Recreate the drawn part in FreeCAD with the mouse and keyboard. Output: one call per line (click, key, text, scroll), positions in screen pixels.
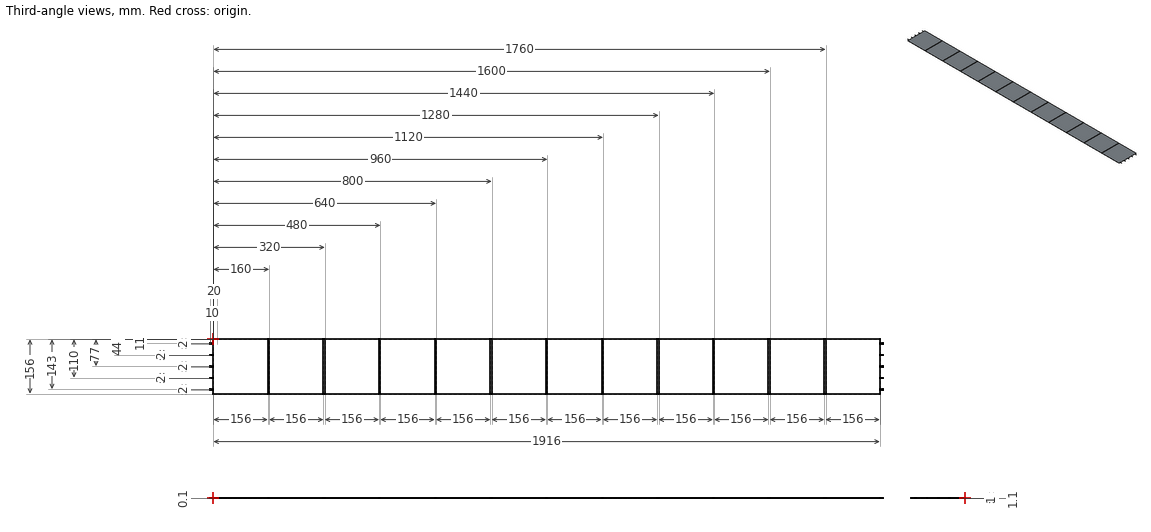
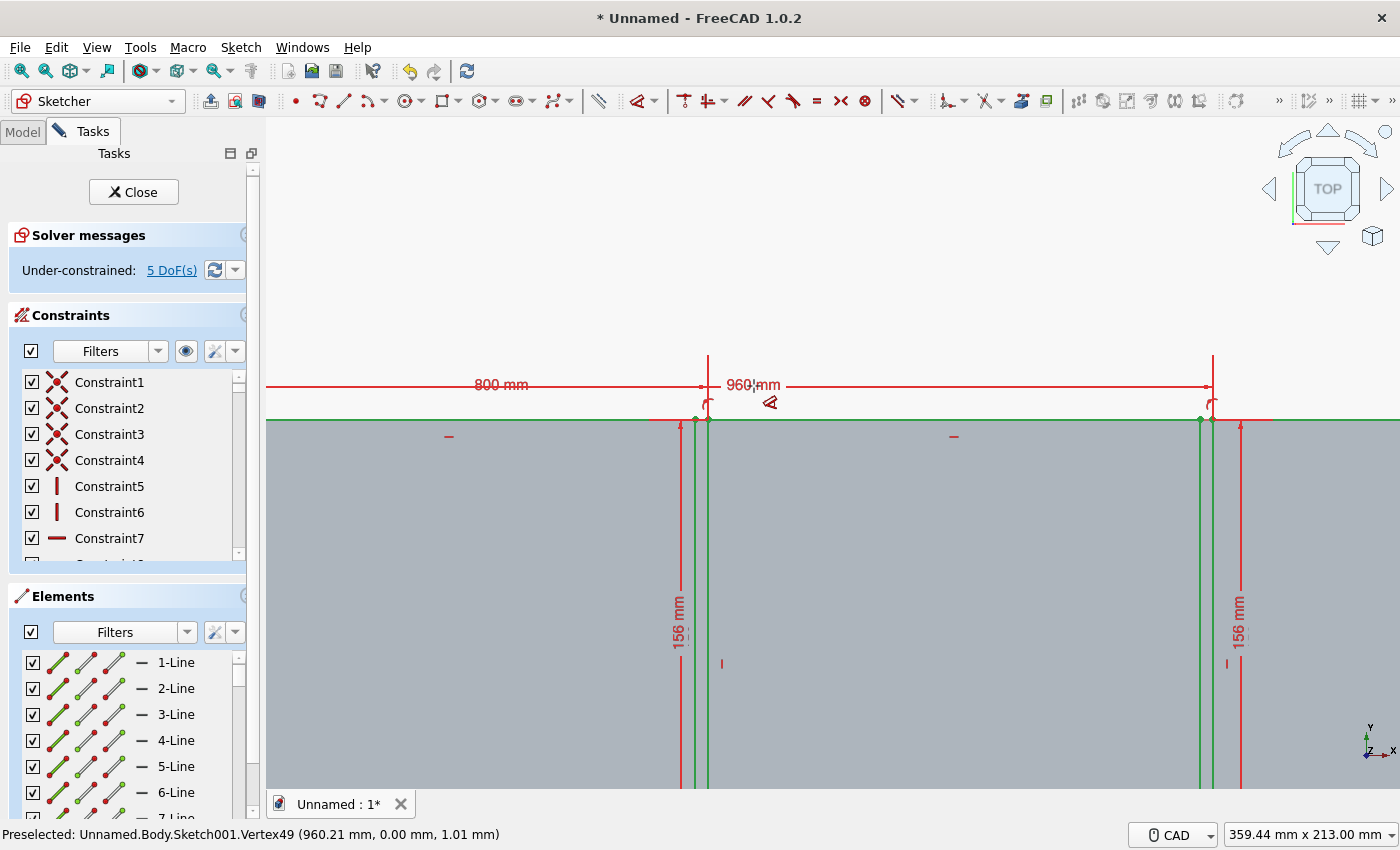
scroll(709, 426, down, 11)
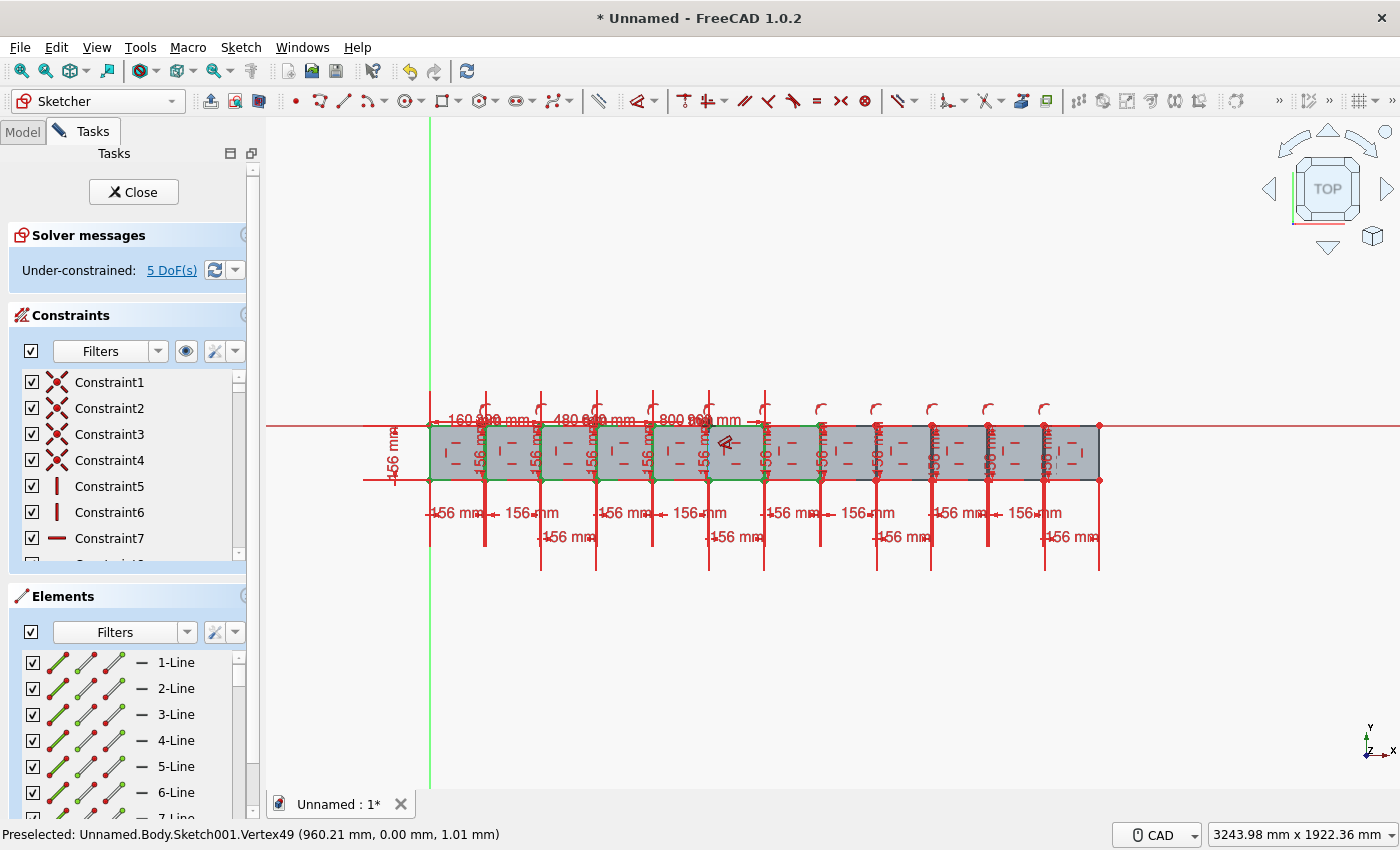
scroll(821, 426, up, 11)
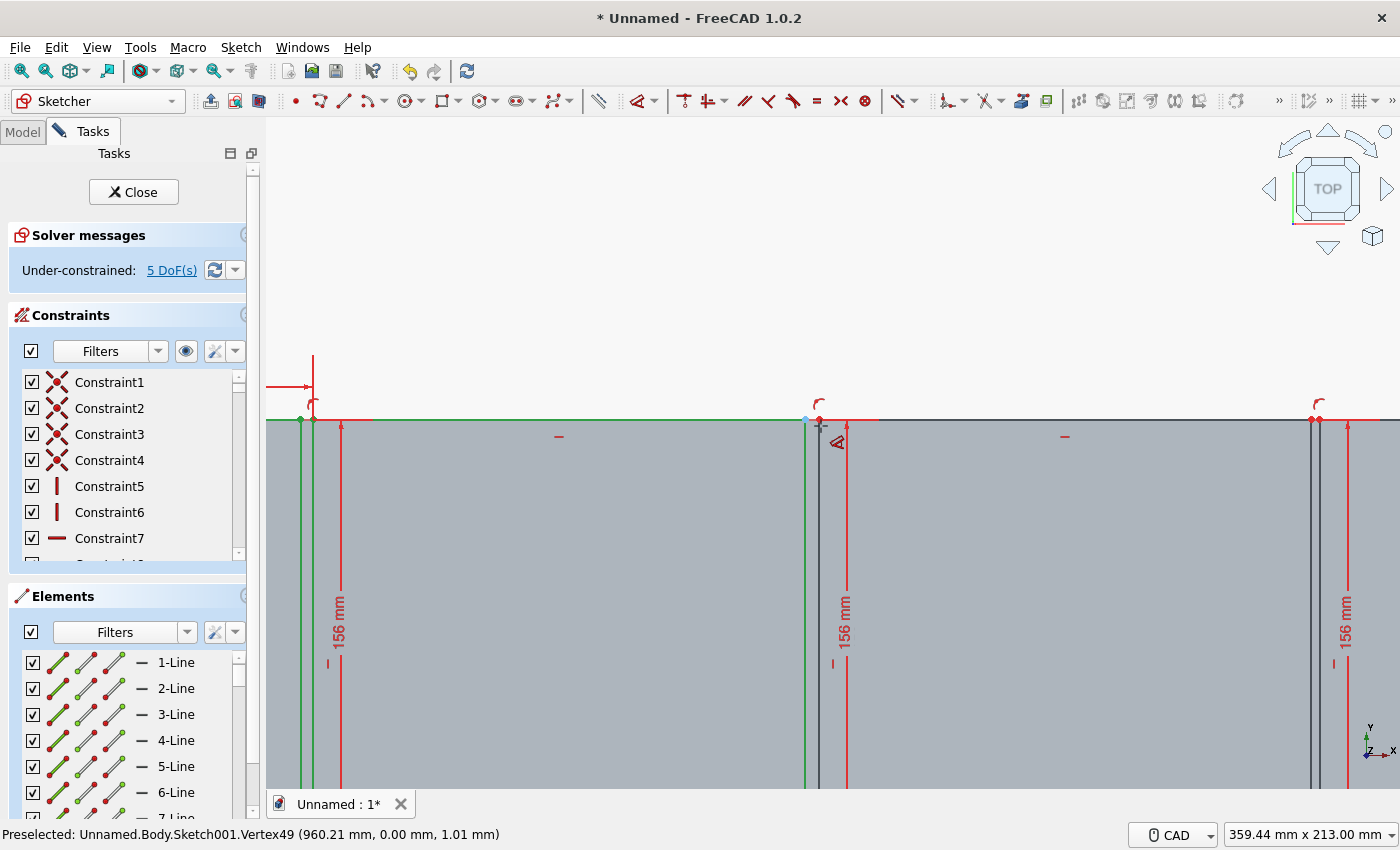
click(819, 420)
click(557, 386)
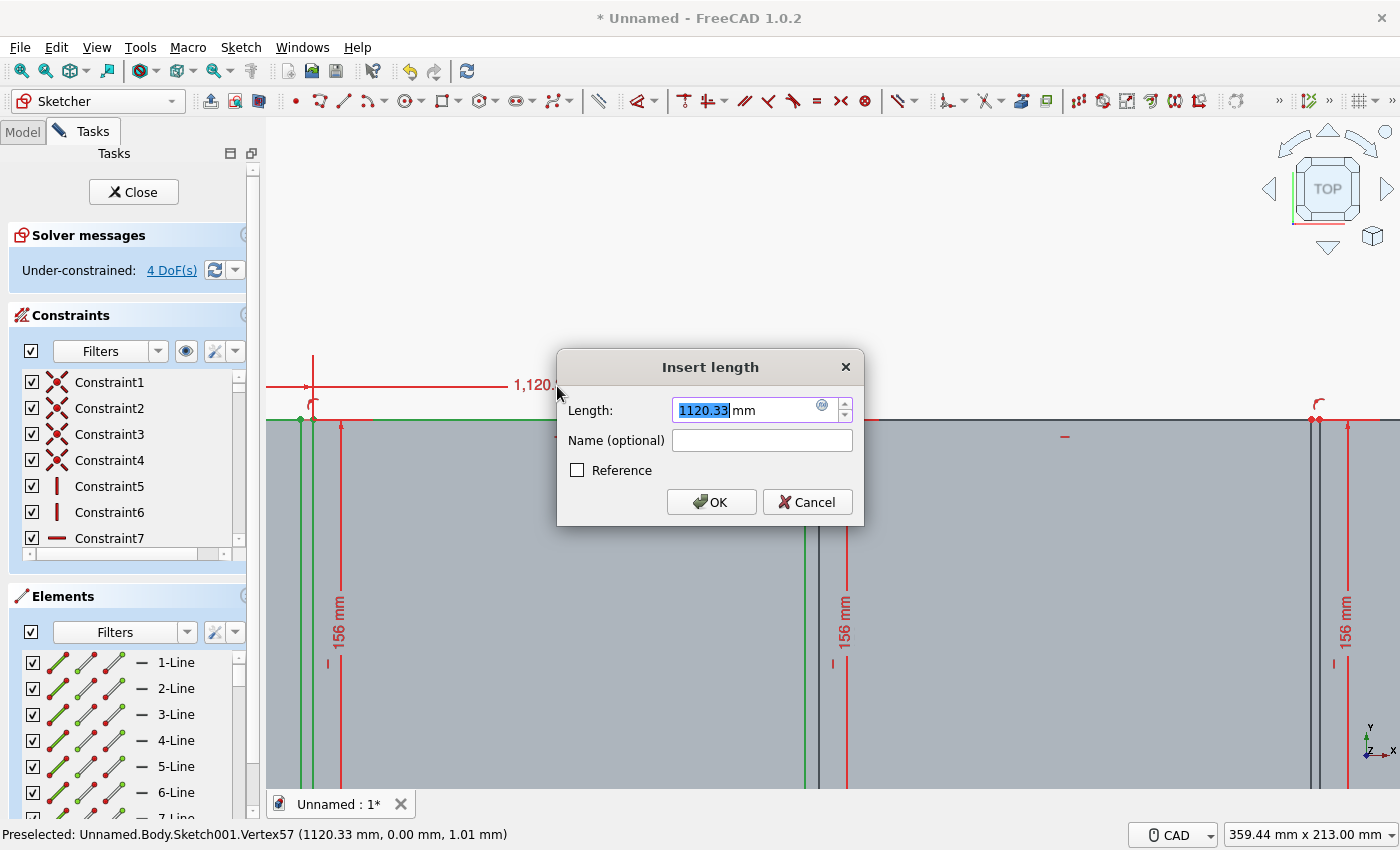
text(1120)
key(Return)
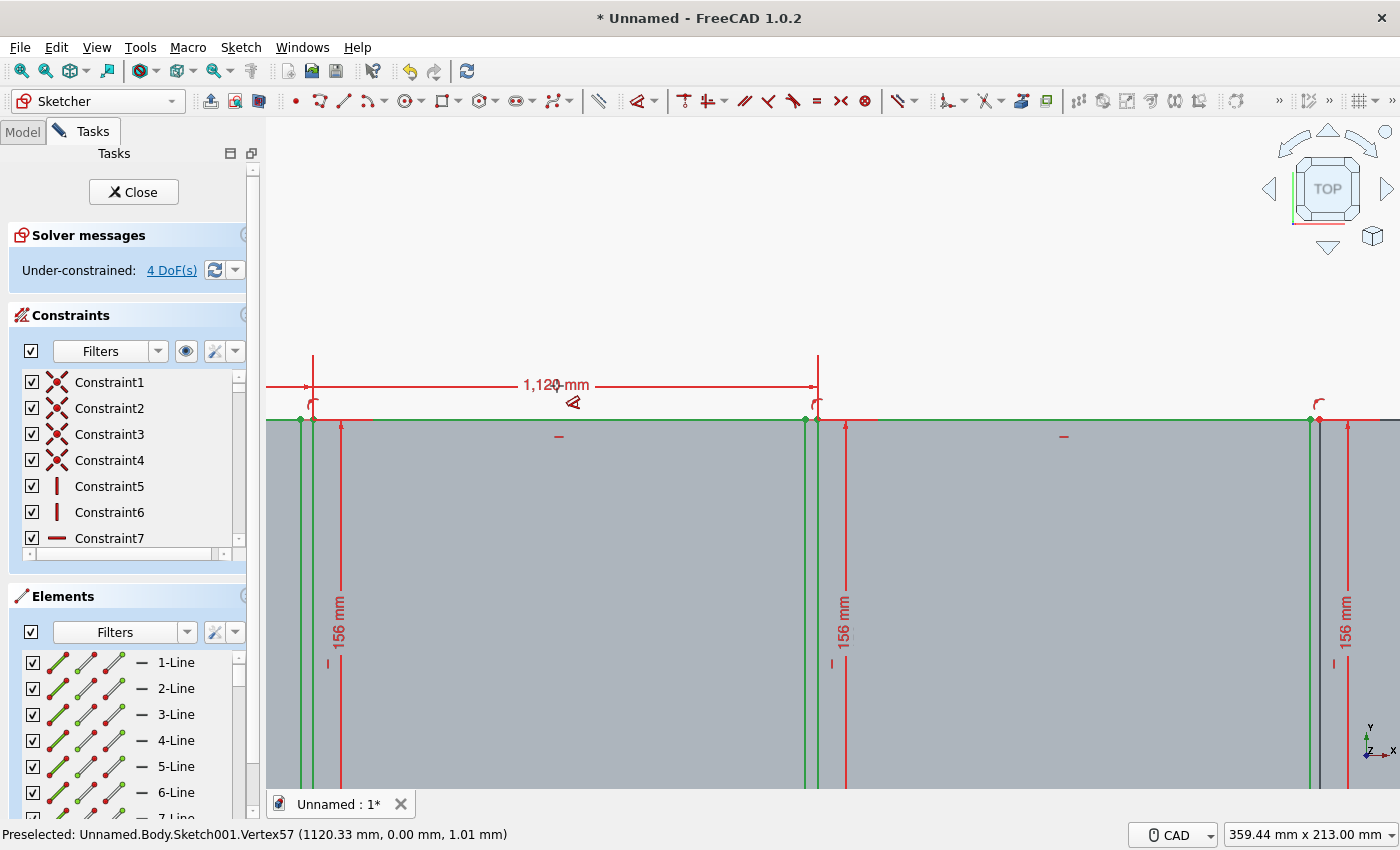
scroll(822, 426, down, 11)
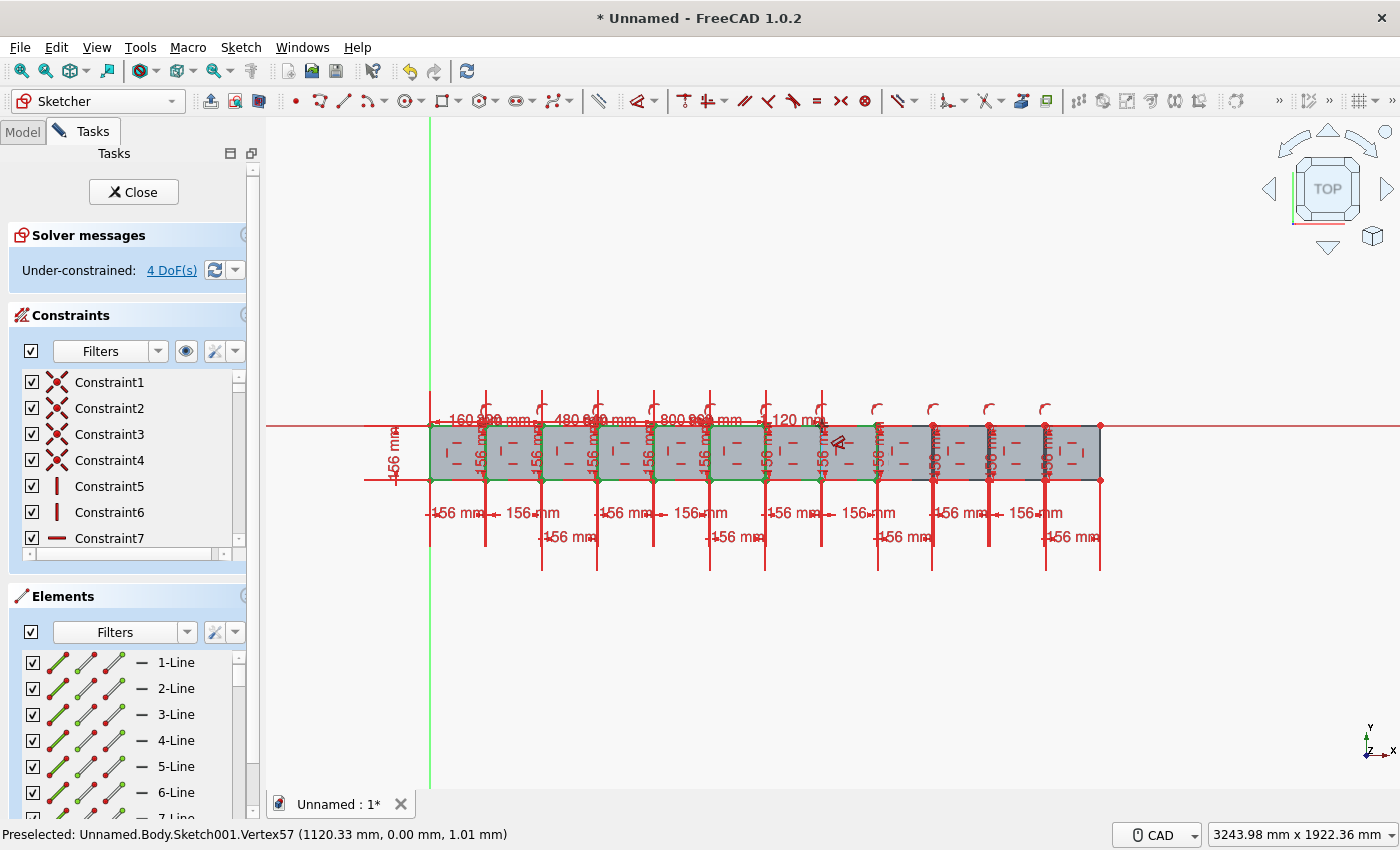
scroll(878, 426, up, 13)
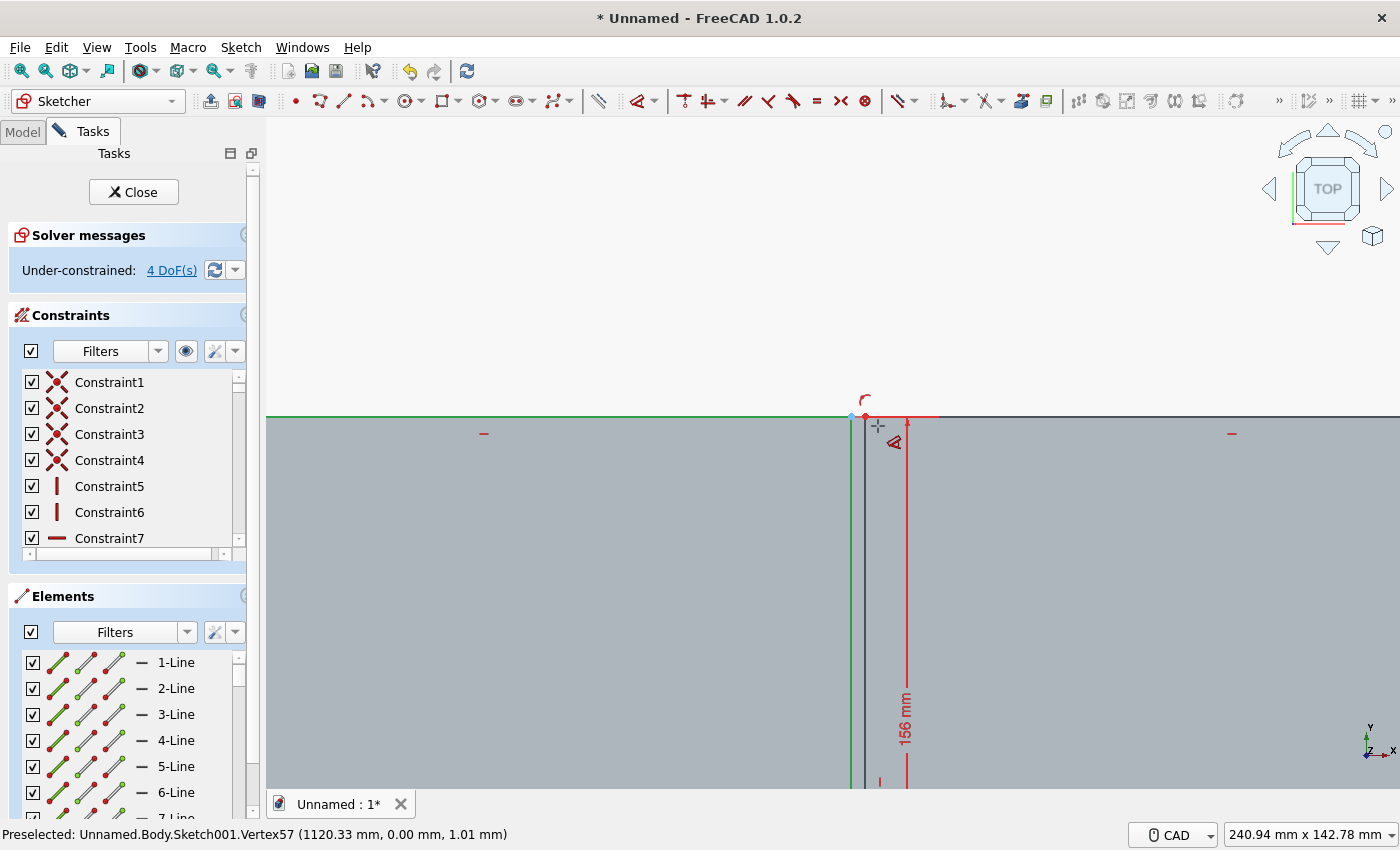
click(865, 417)
click(580, 383)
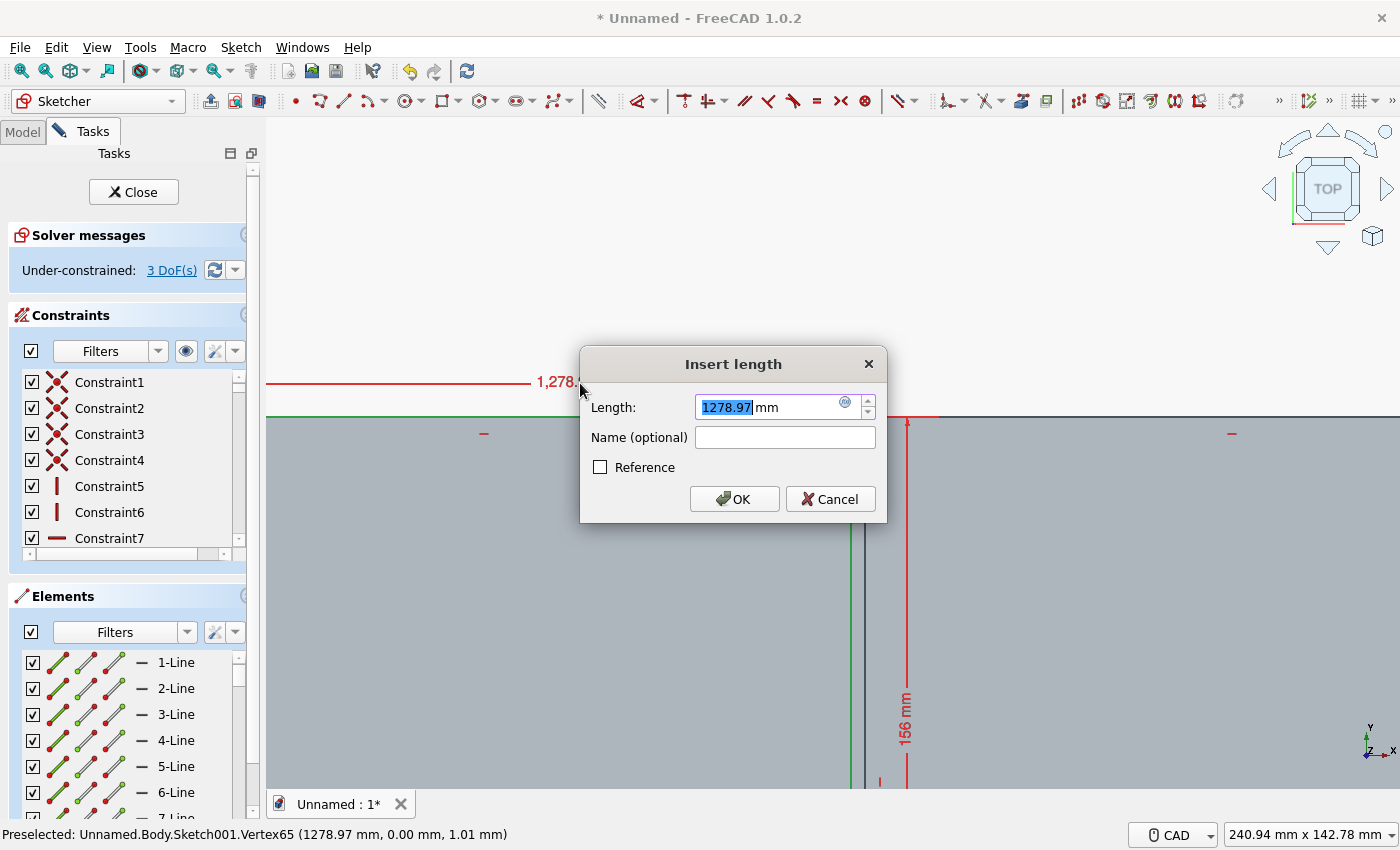
text(1280)
key(Return)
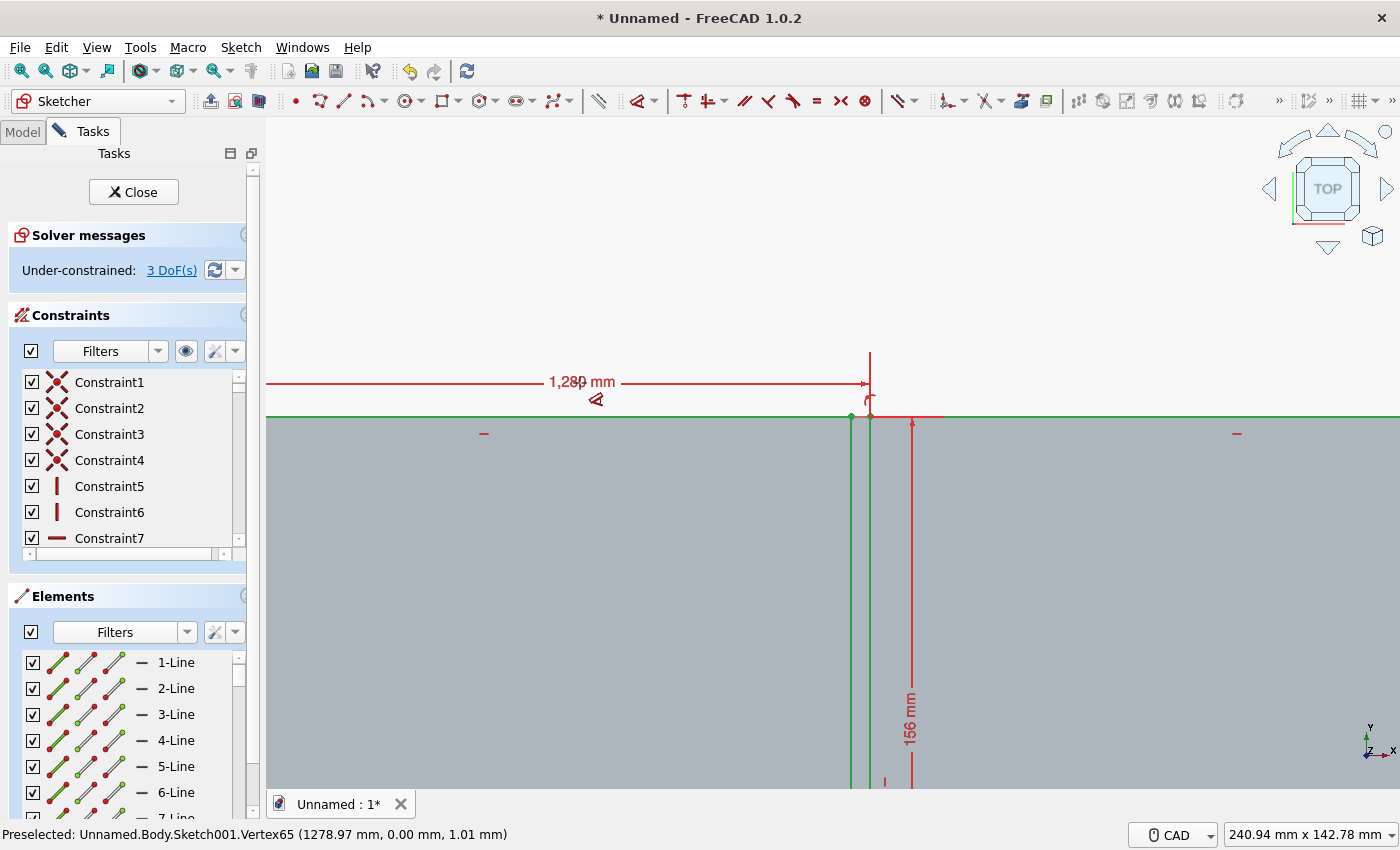
scroll(878, 426, down, 13)